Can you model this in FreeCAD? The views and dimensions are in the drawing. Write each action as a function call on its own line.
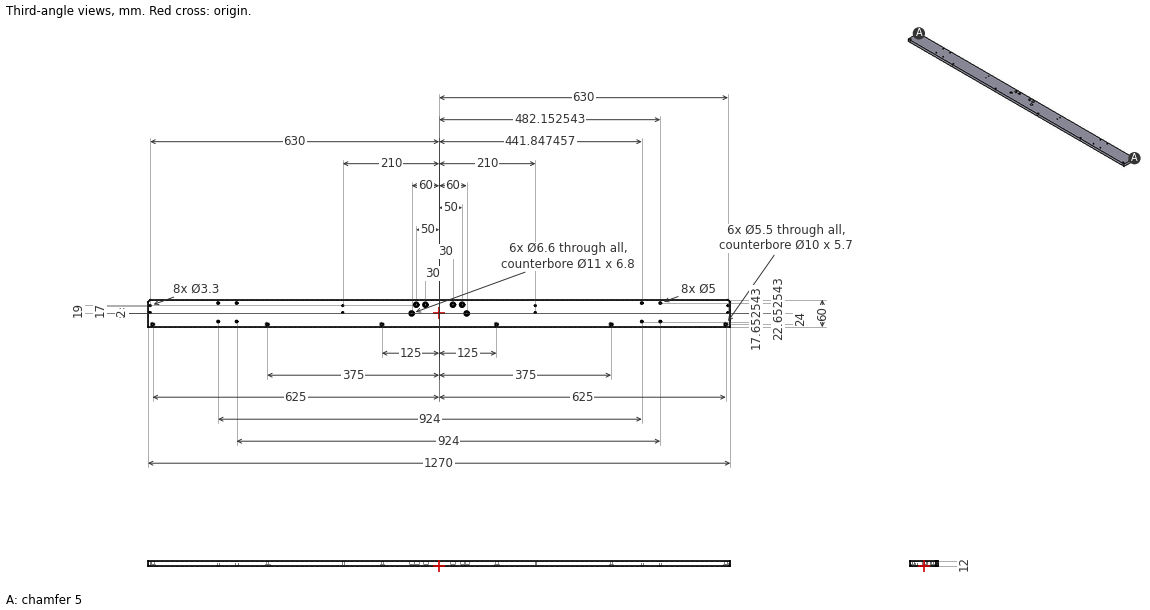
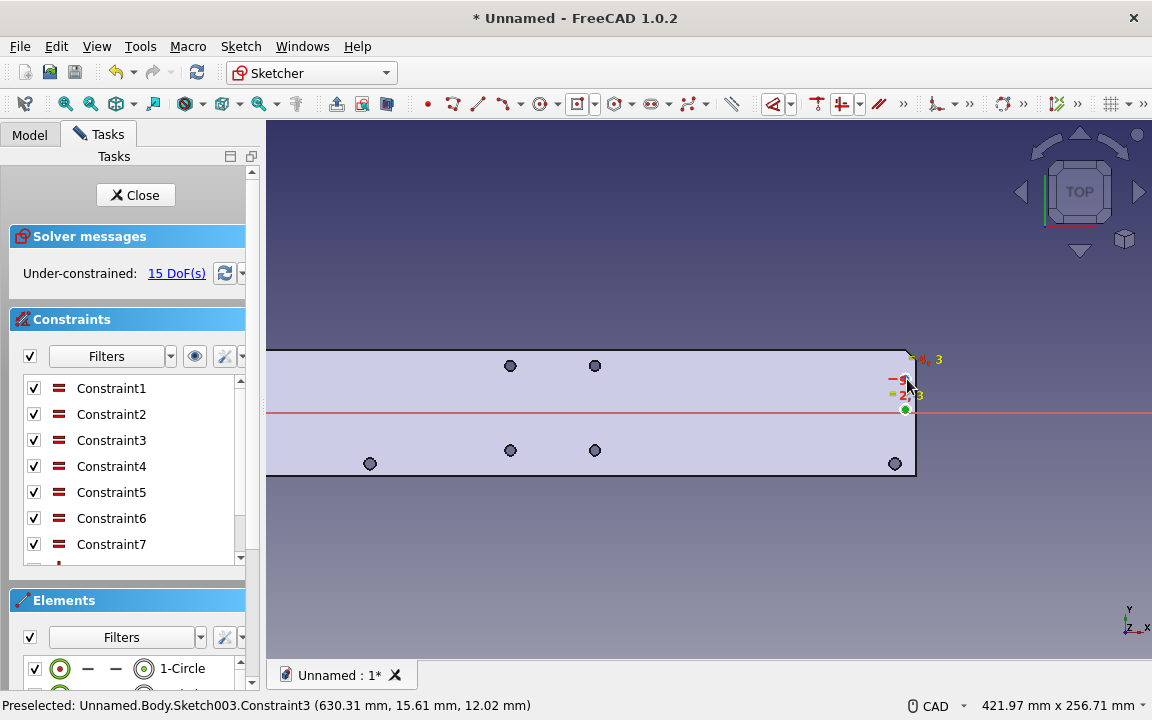
scroll(905, 379, up, 4)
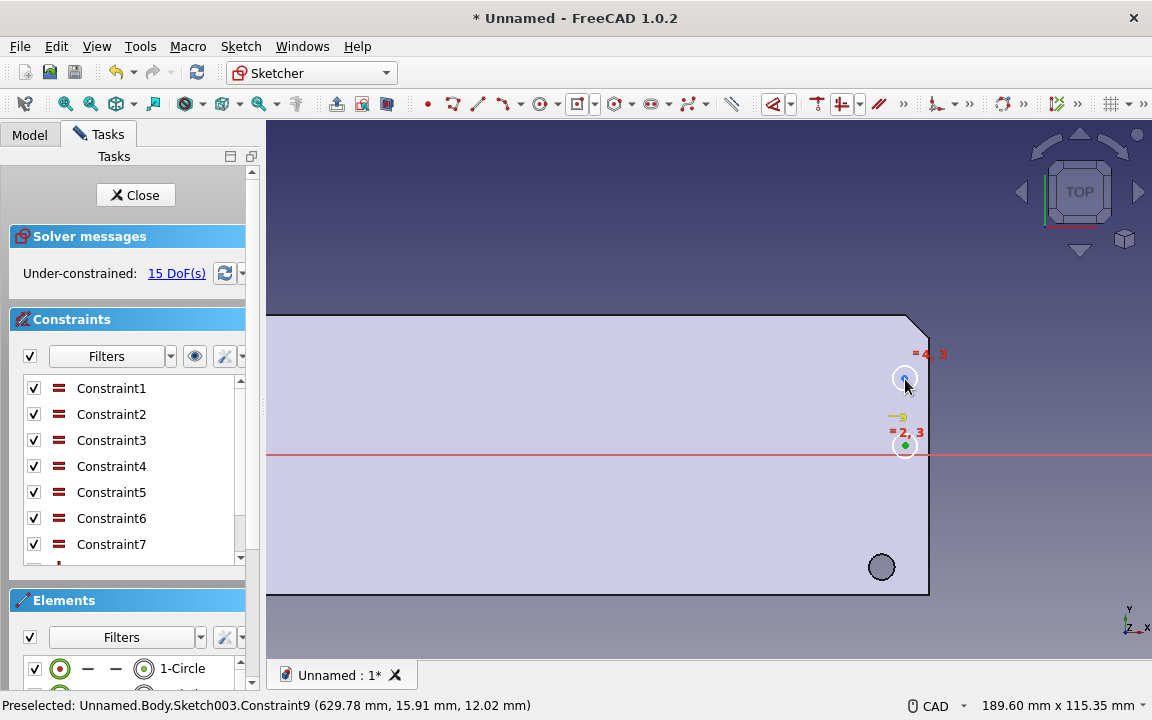
click(905, 378)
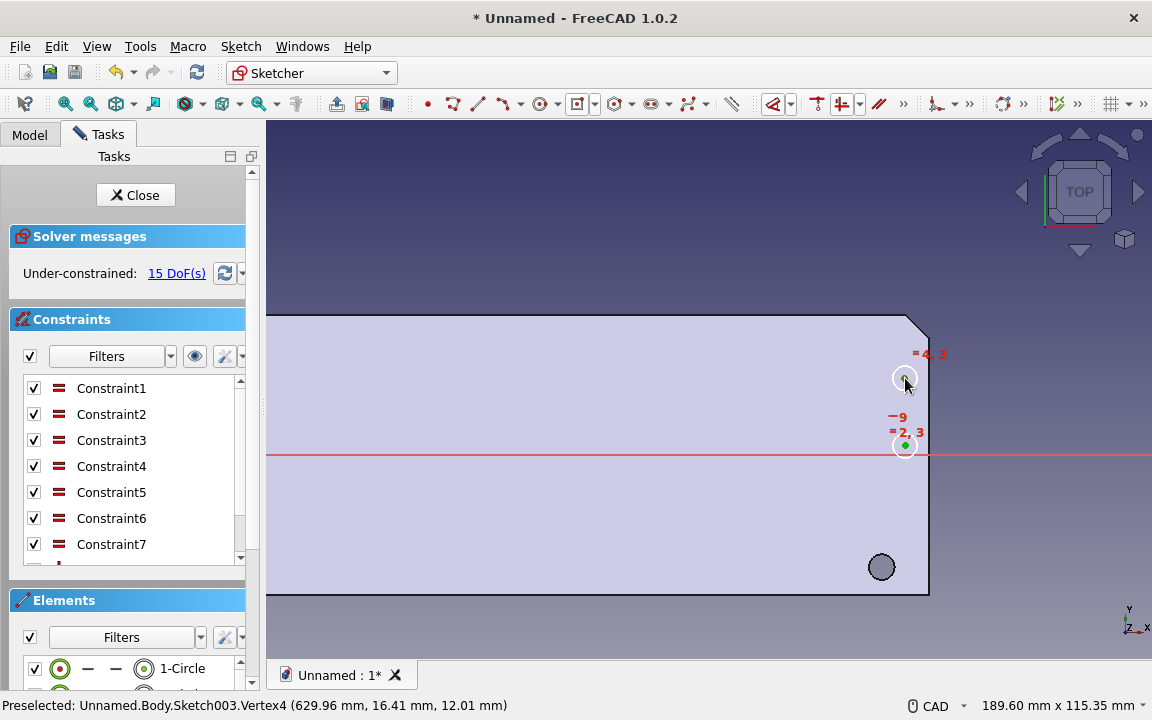
click(860, 104)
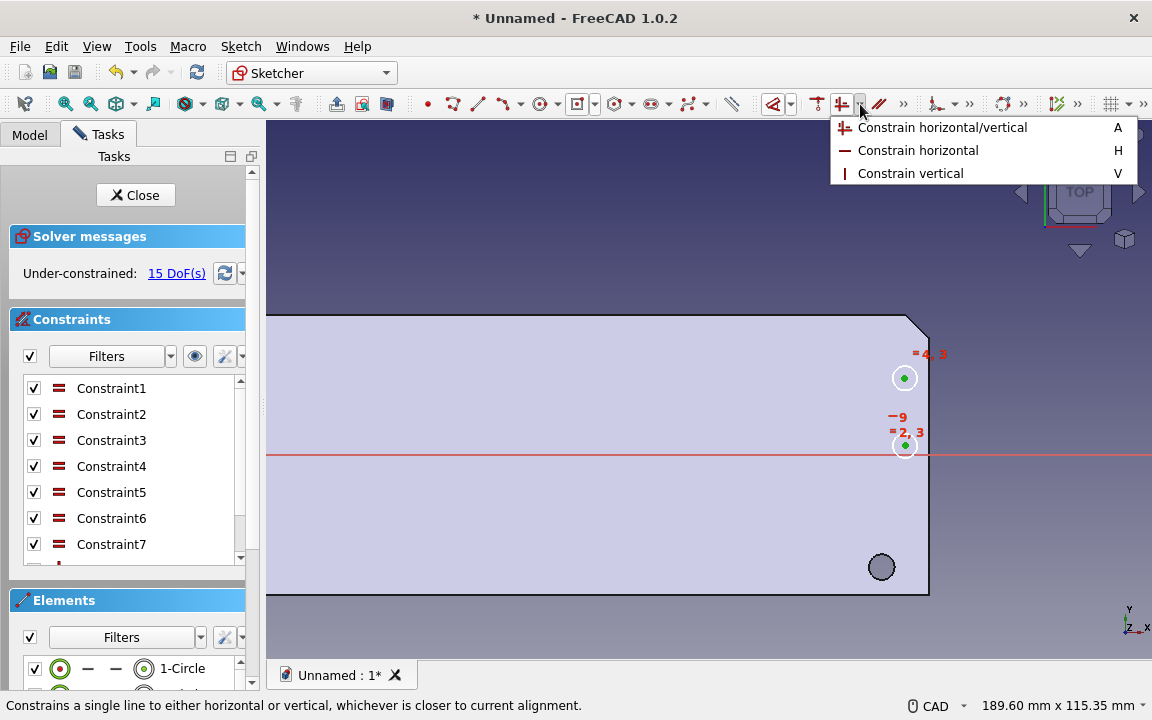
click(984, 174)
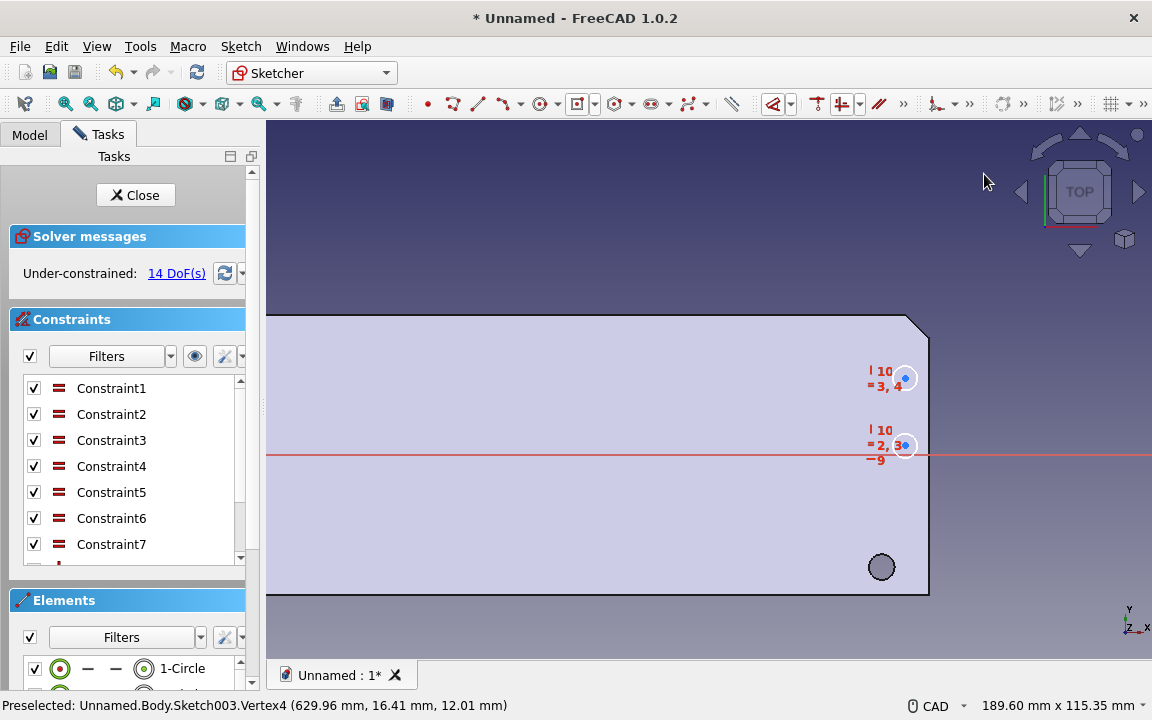
scroll(908, 387, down, 12)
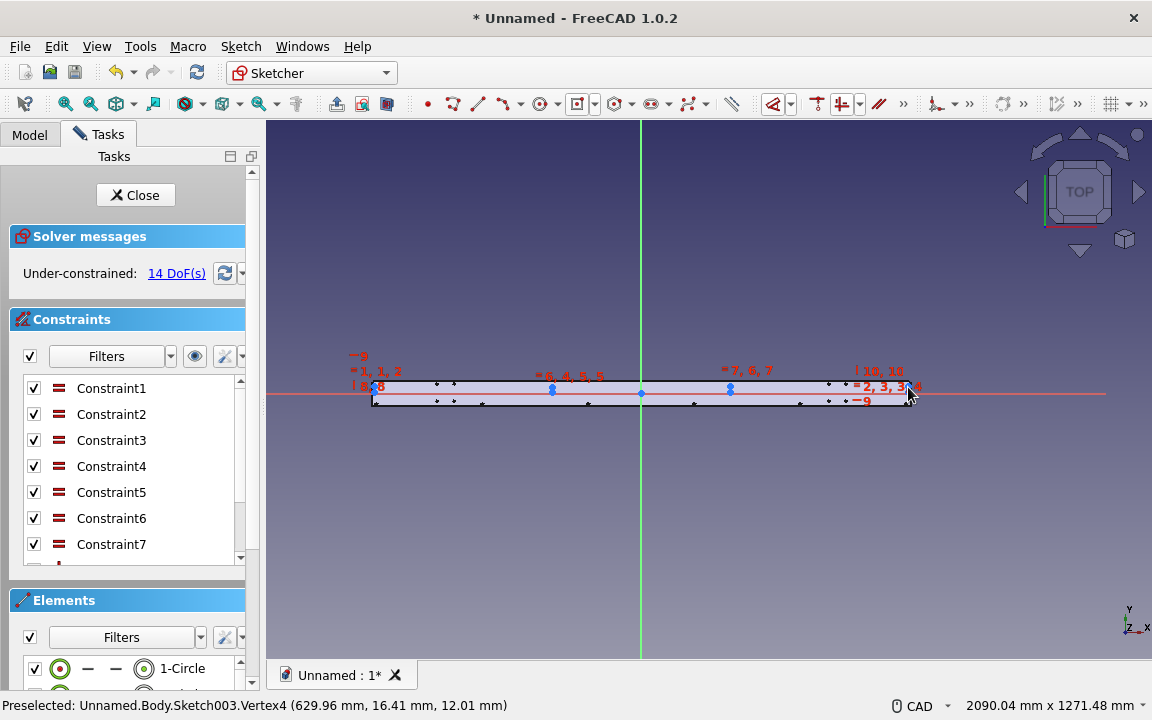
scroll(374, 387, up, 4)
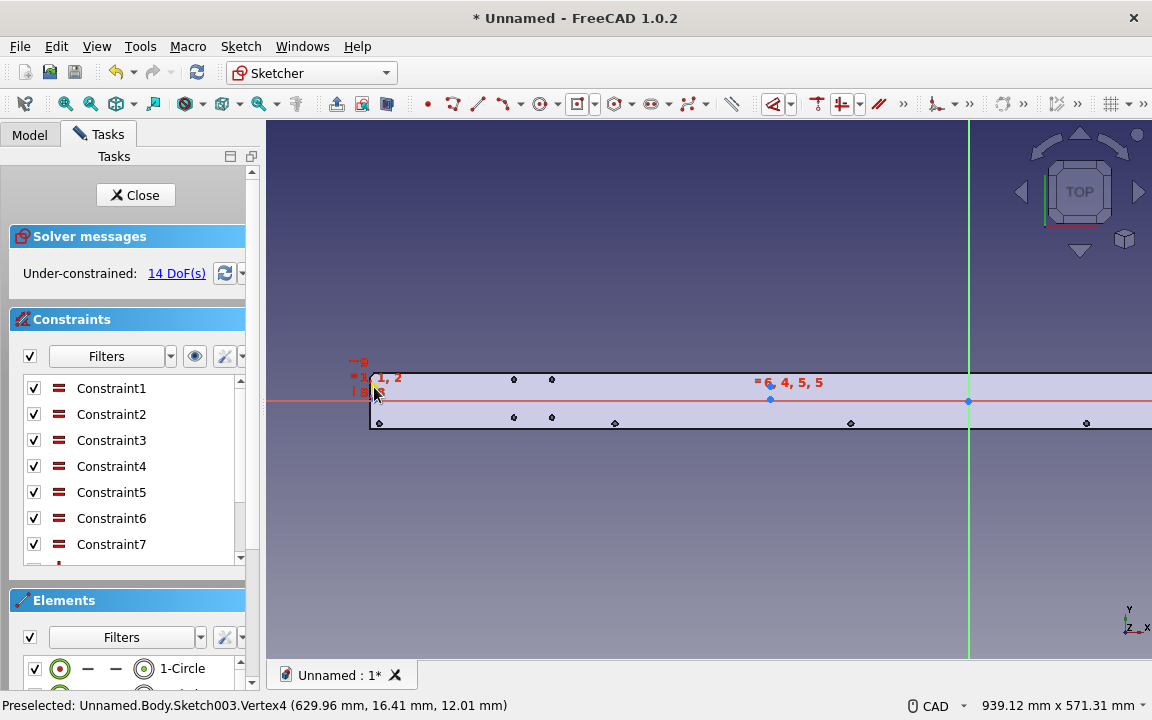
click(374, 386)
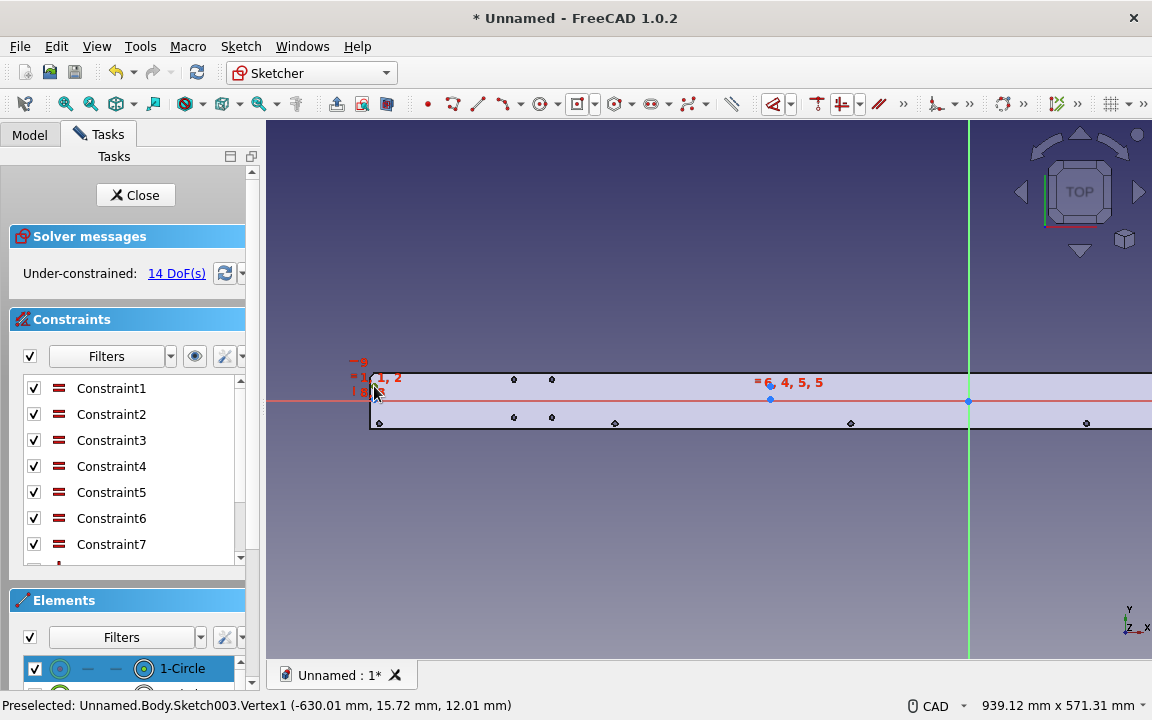
scroll(373, 387, down, 4)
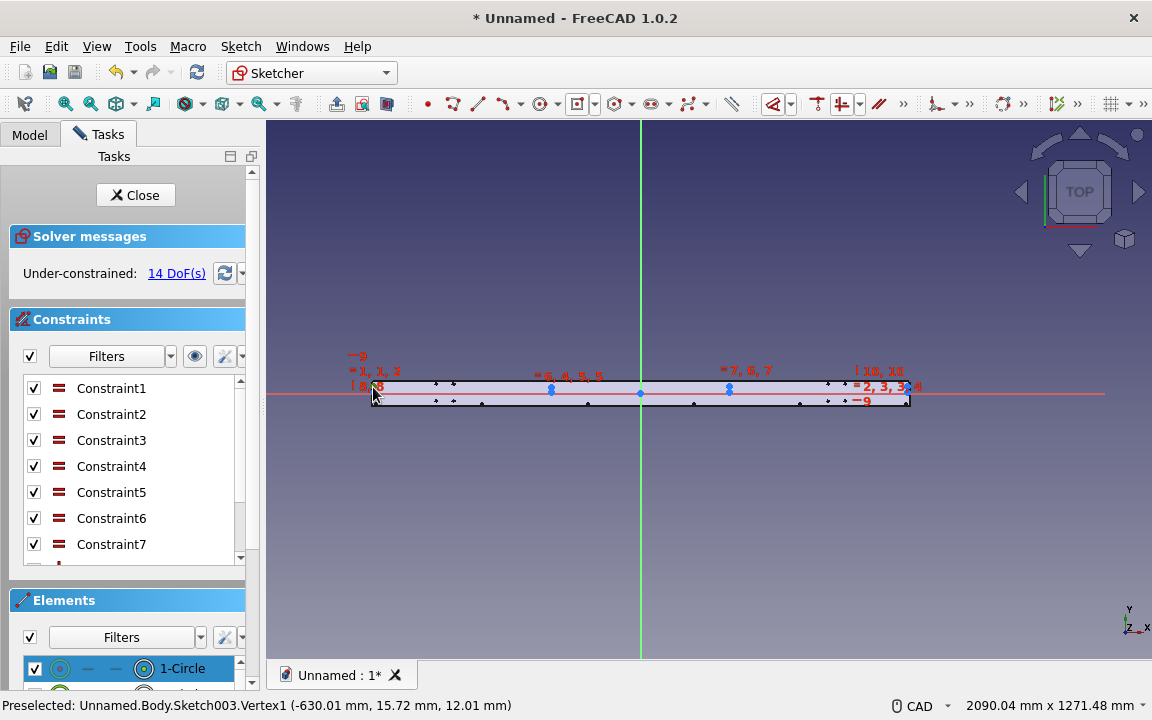
scroll(908, 387, up, 4)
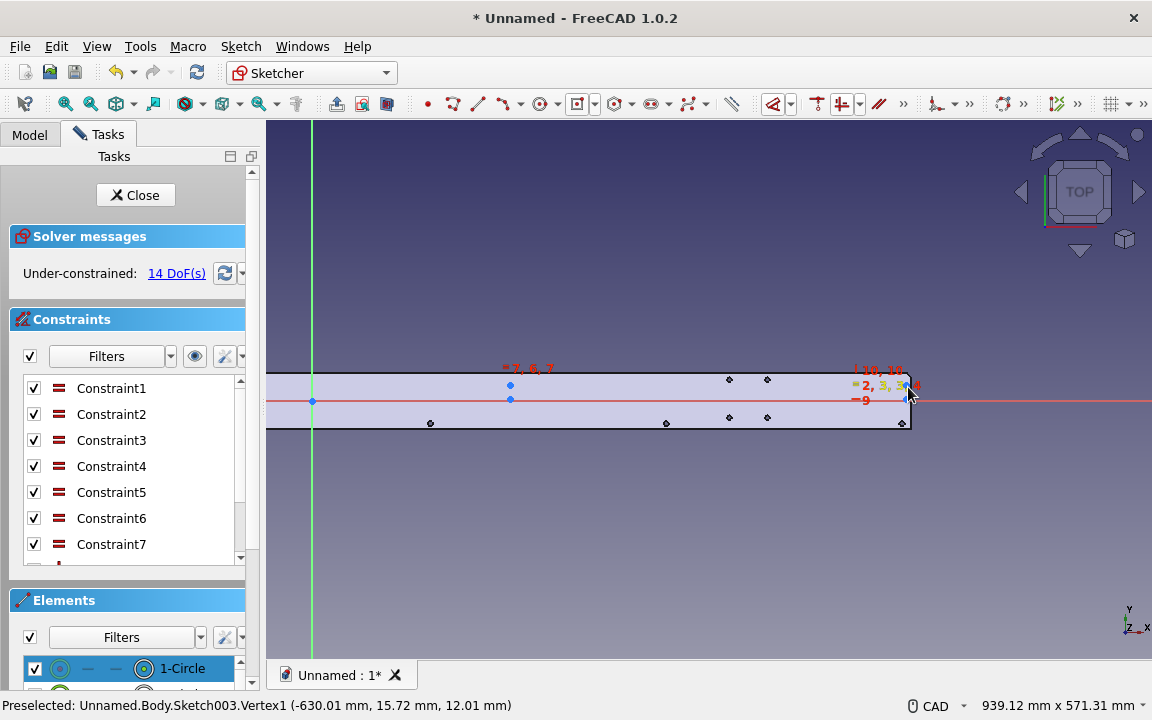
scroll(907, 386, up, 4)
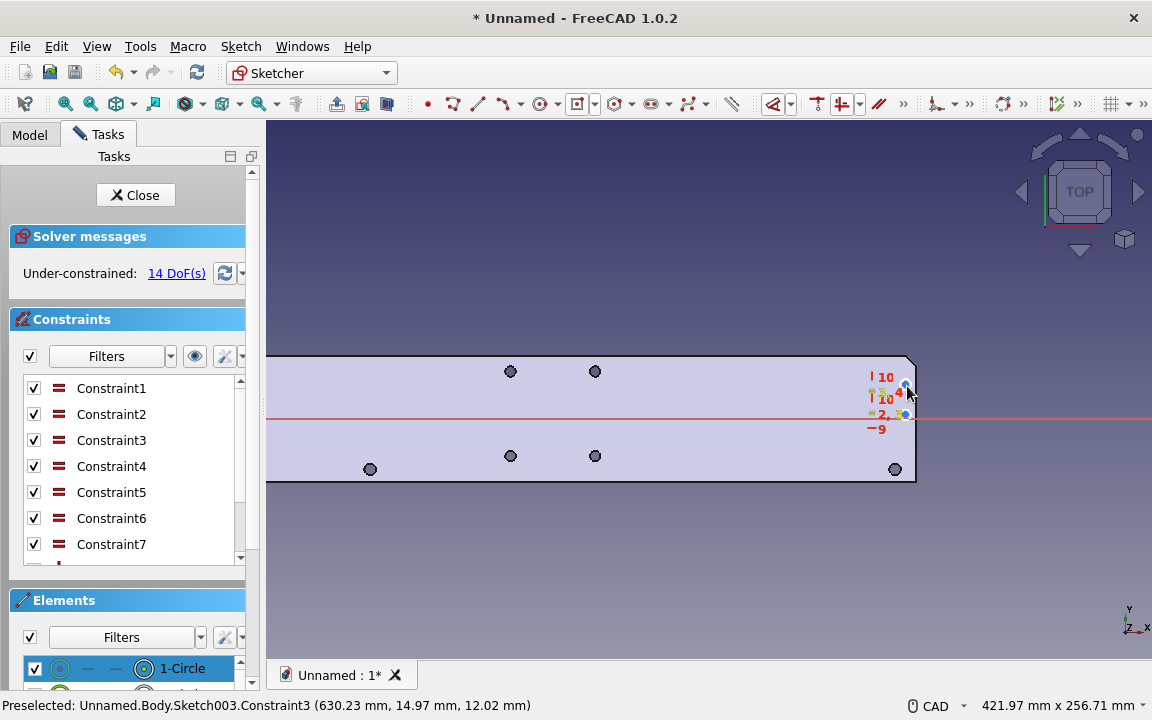
click(906, 385)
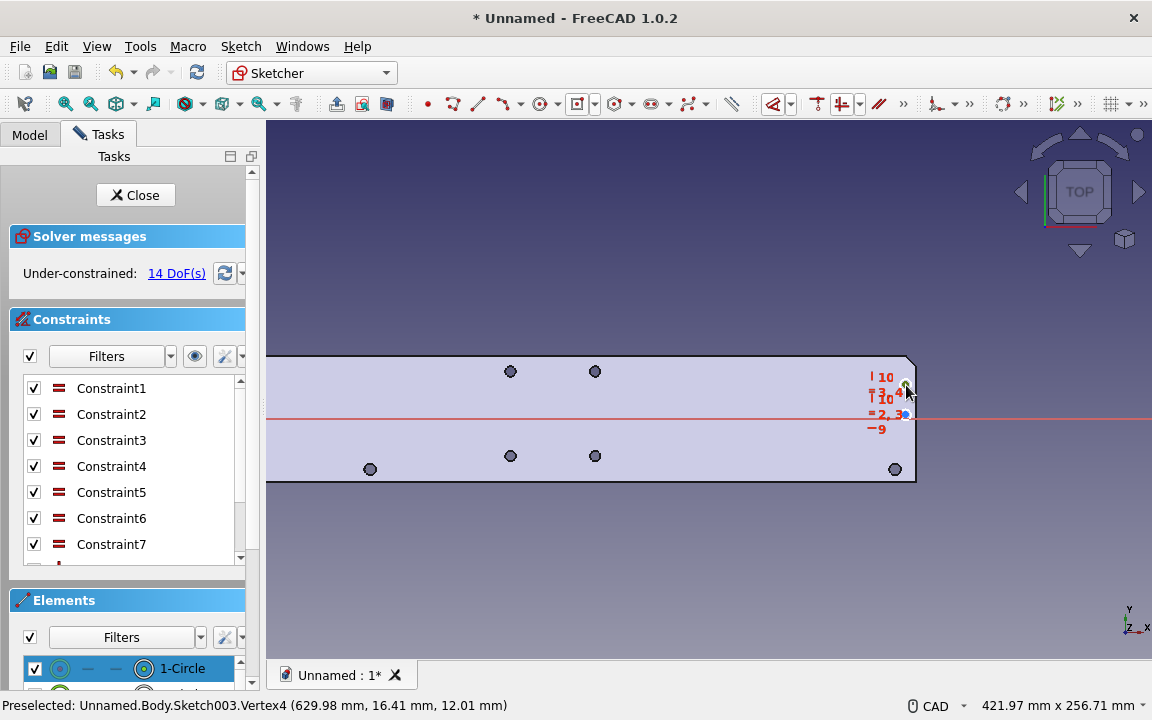
key(h)